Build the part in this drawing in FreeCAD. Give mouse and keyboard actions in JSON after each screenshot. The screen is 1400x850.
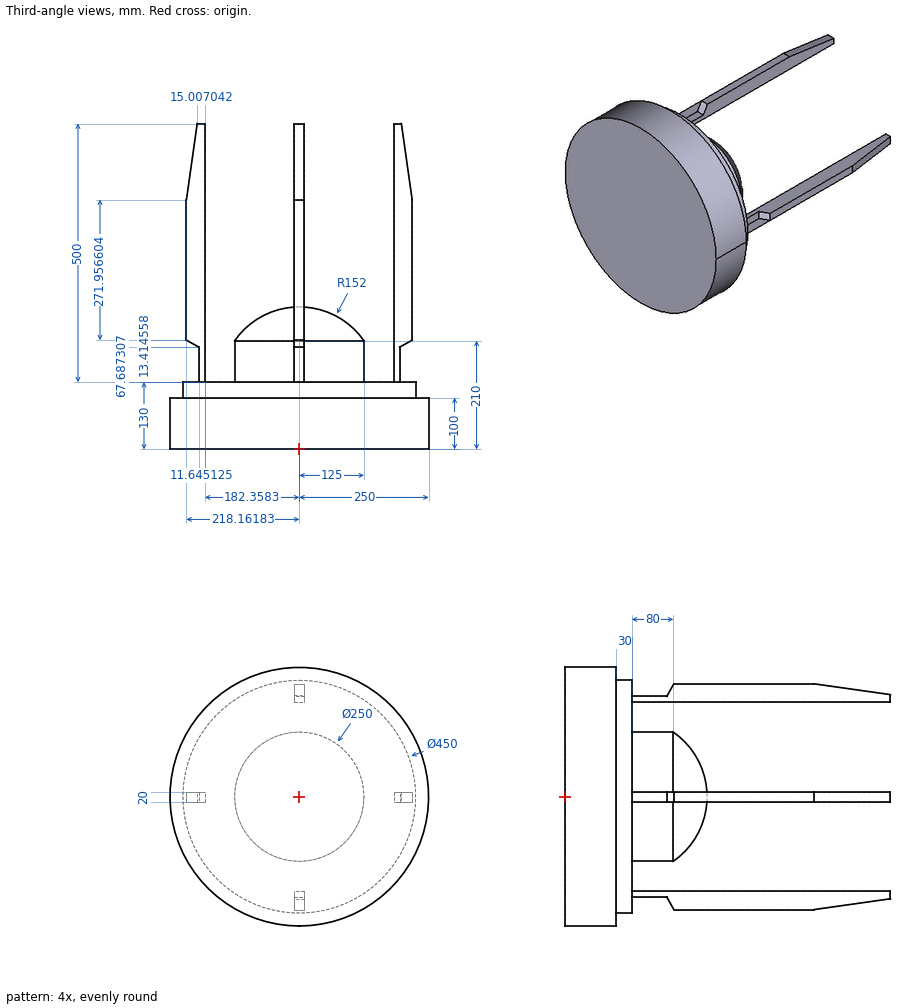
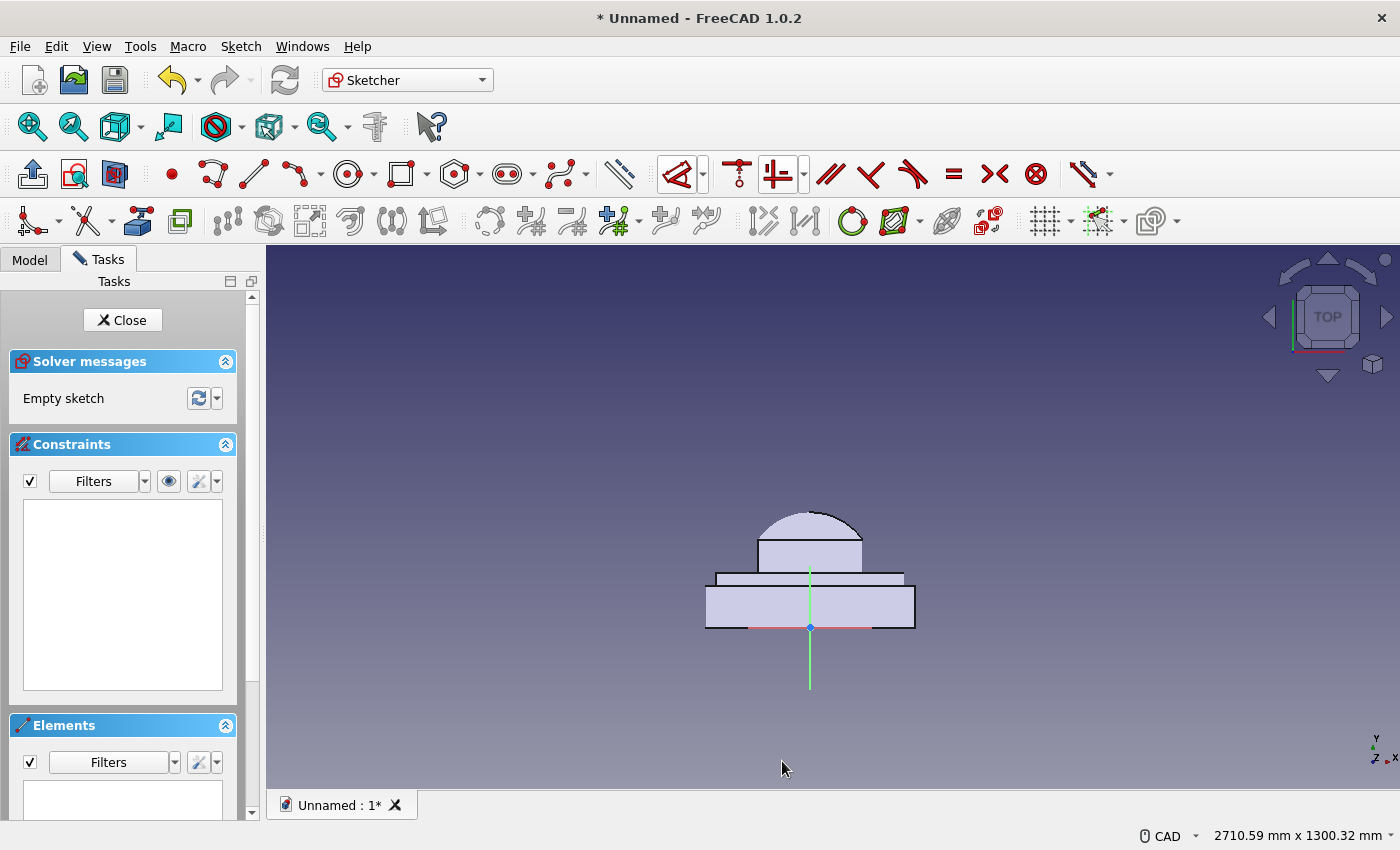
{"action": "left_click", "coordinate": [213, 174]}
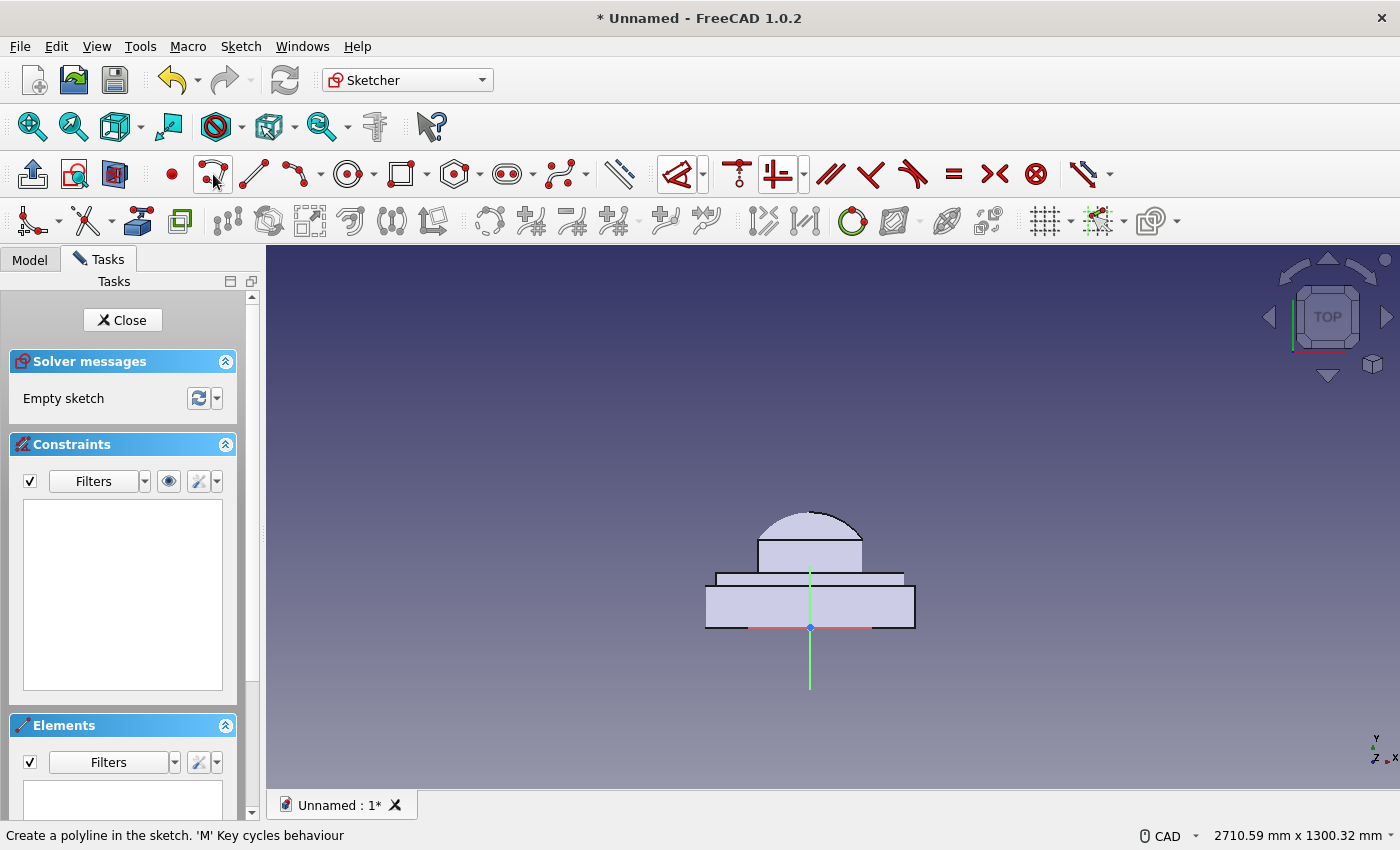
{"action": "left_click", "coordinate": [734, 573]}
{"action": "left_click", "coordinate": [734, 364]}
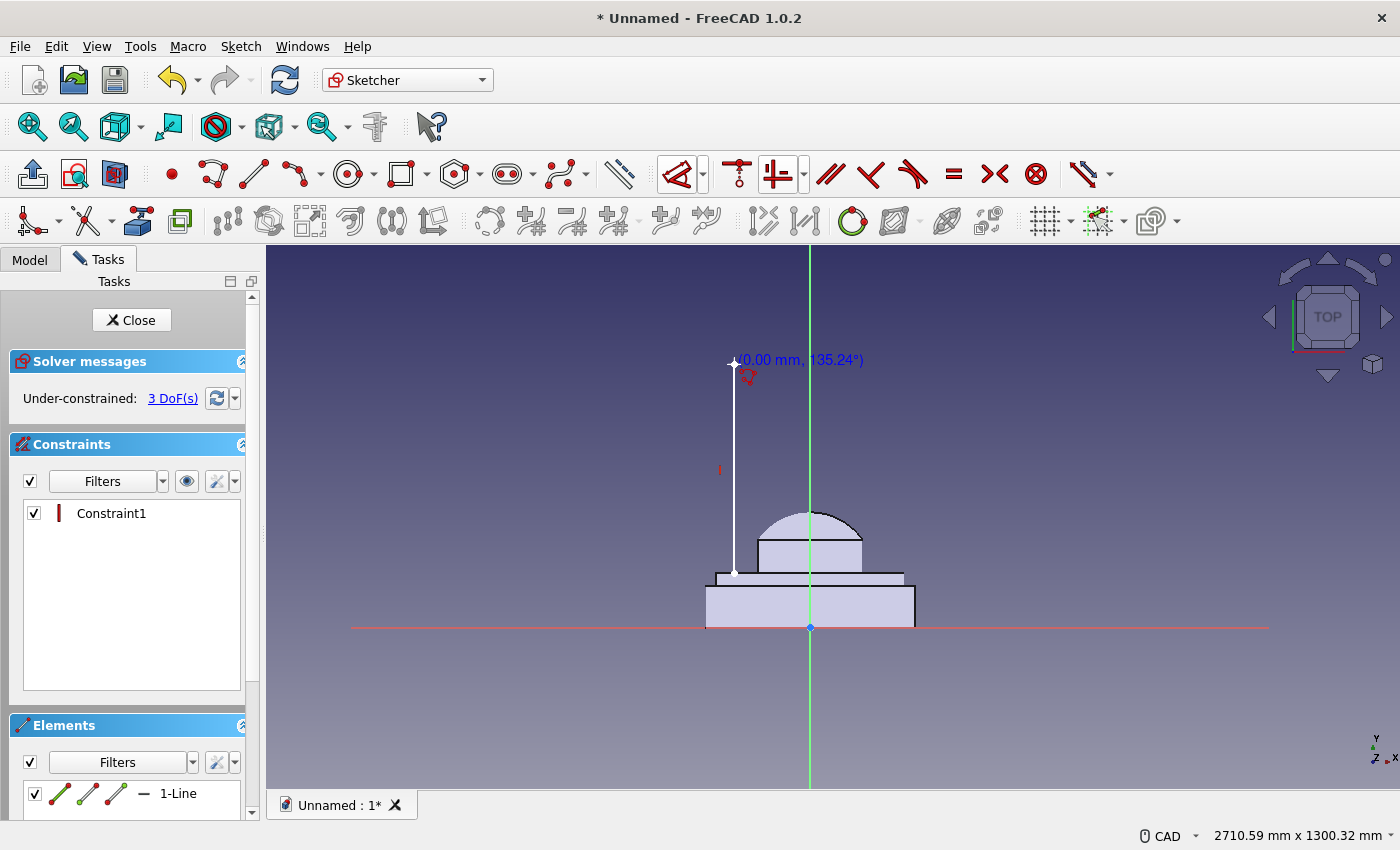
{"action": "scroll", "coordinate": [728, 364], "scroll_direction": "up", "scroll_amount": 5}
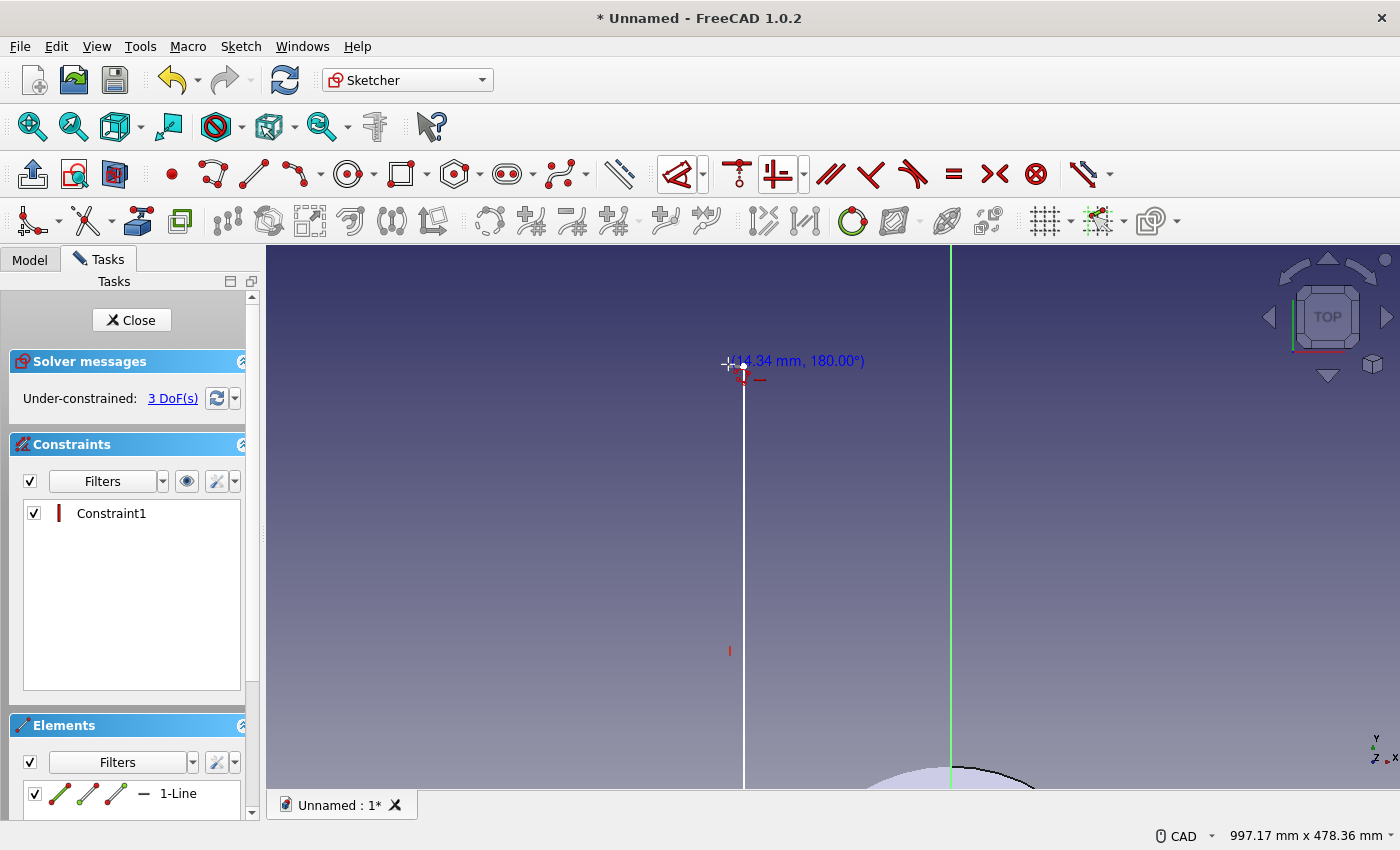
{"action": "left_click", "coordinate": [726, 364]}
{"action": "left_click", "coordinate": [703, 531]}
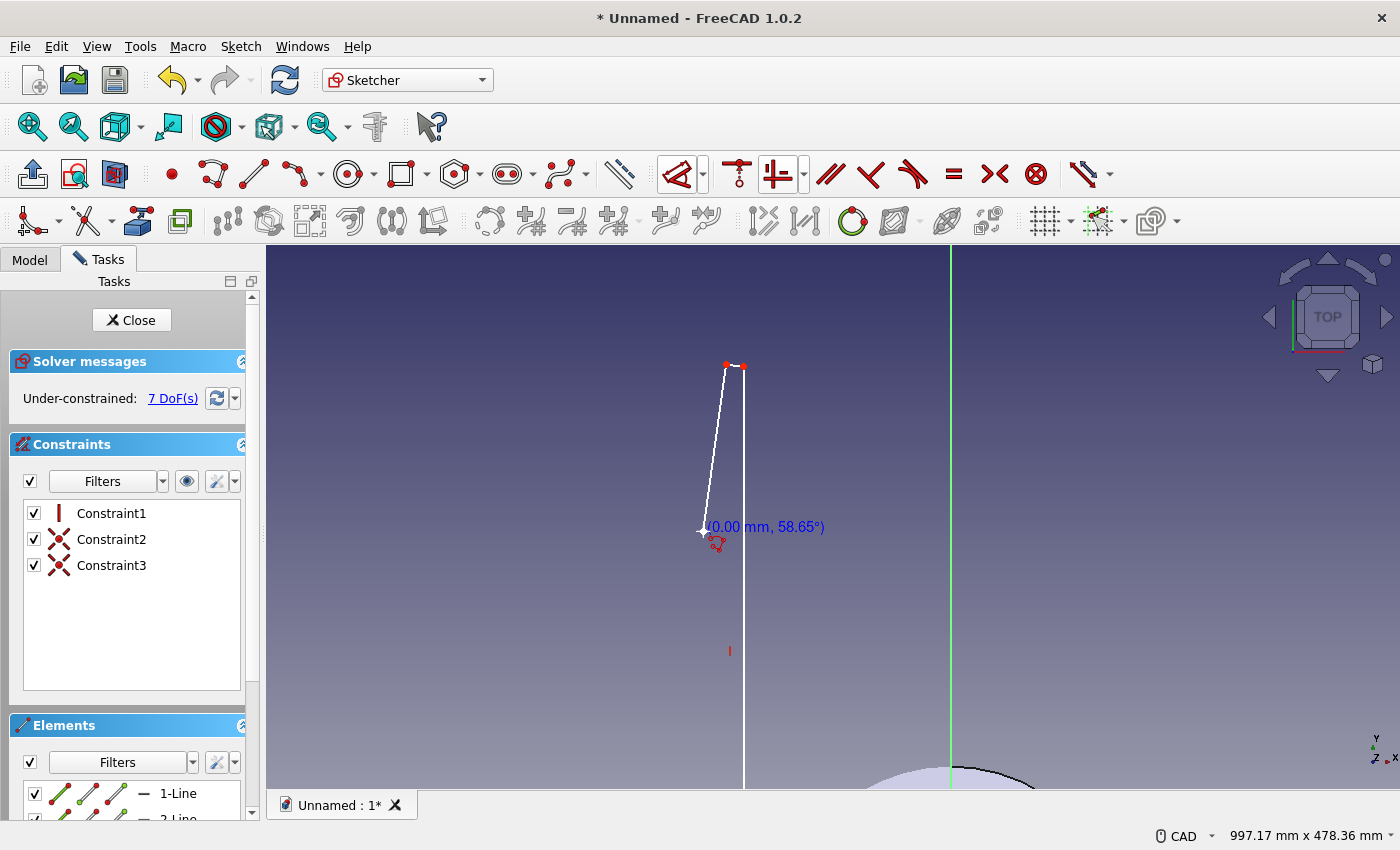
{"action": "scroll", "coordinate": [714, 350], "scroll_direction": "down", "scroll_amount": 4}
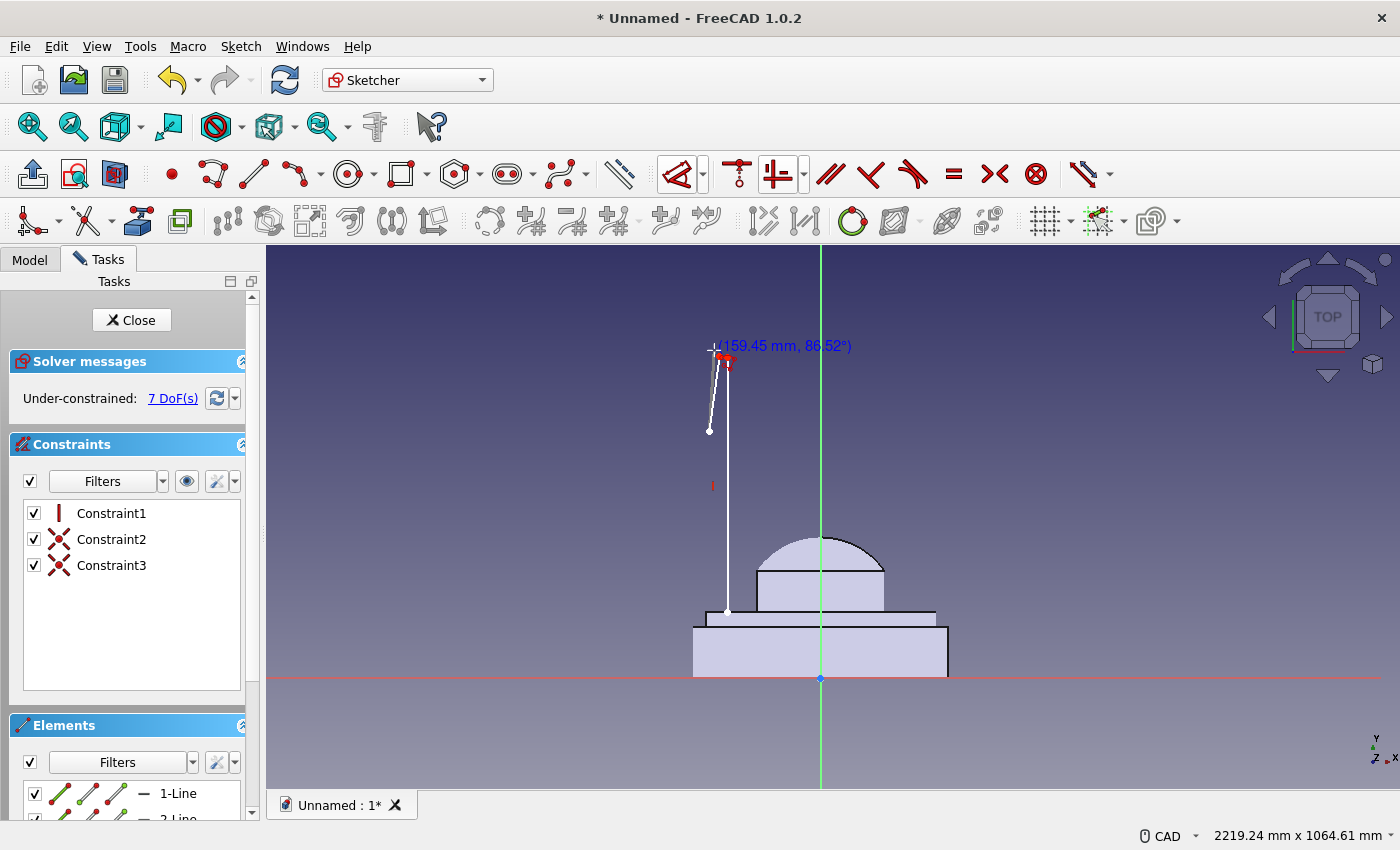
{"action": "left_click", "coordinate": [709, 570]}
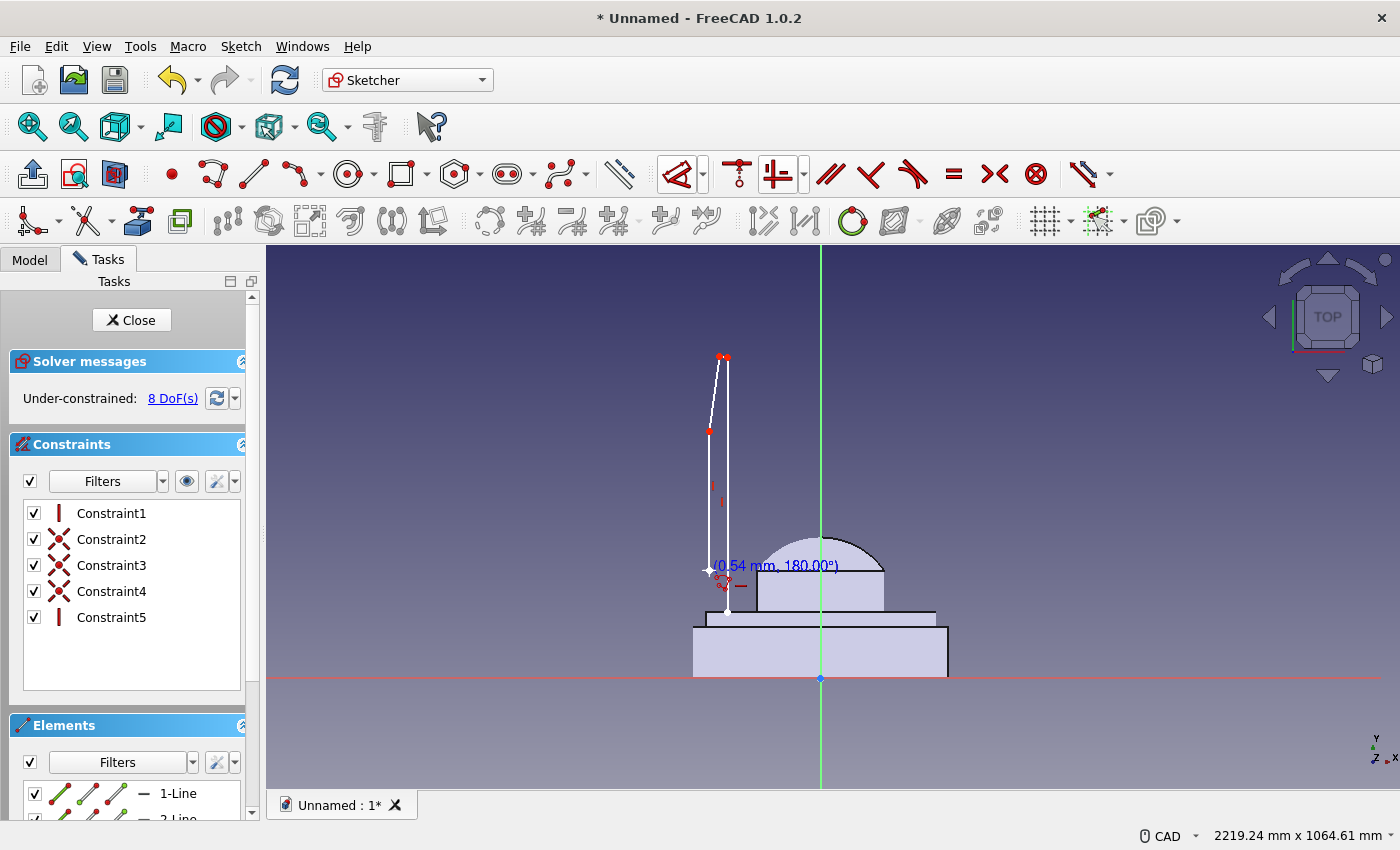
{"action": "scroll", "coordinate": [721, 577], "scroll_direction": "up", "scroll_amount": 5}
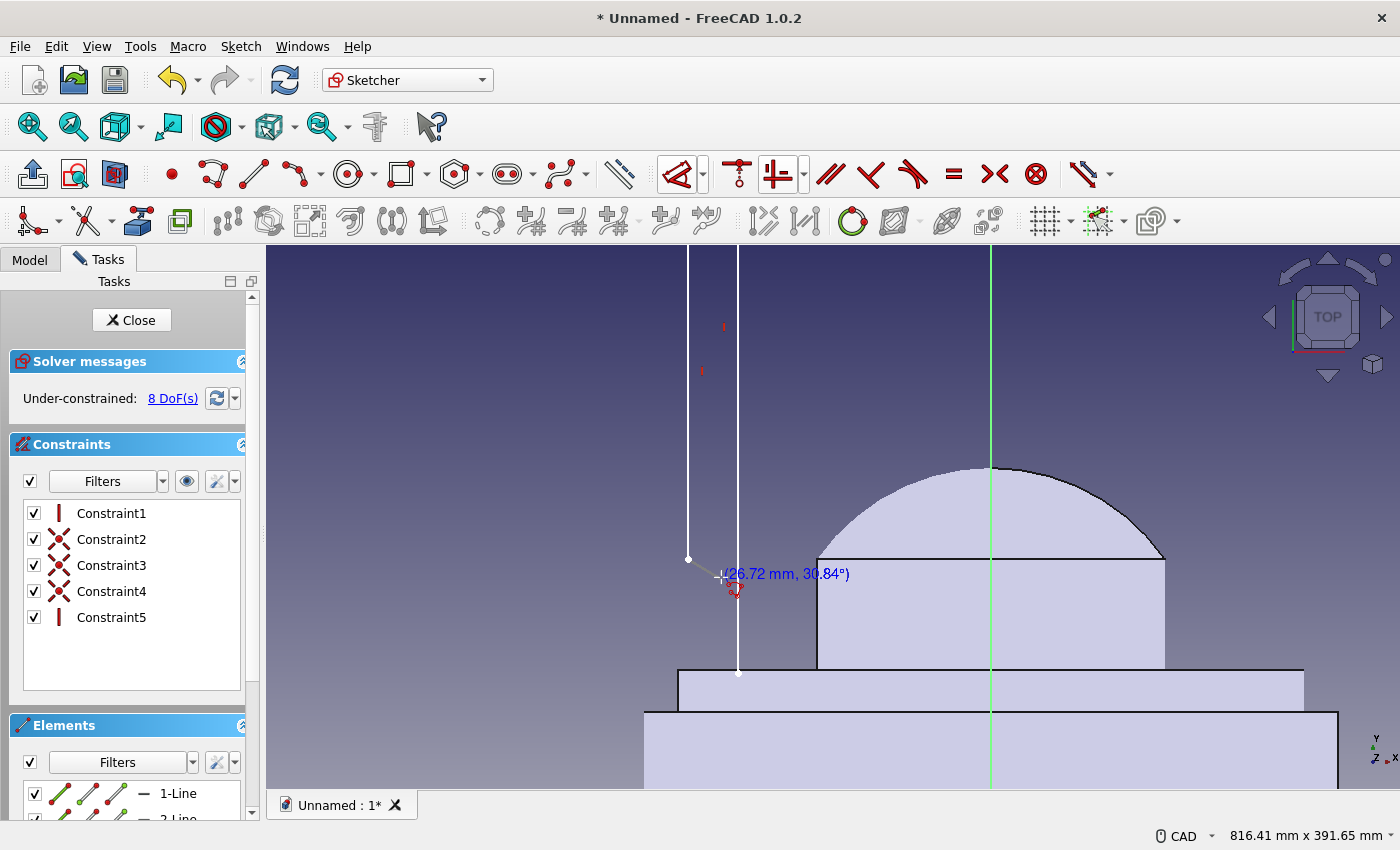
{"action": "left_click", "coordinate": [722, 576]}
{"action": "left_click", "coordinate": [722, 670]}
{"action": "left_click", "coordinate": [738, 673]}
{"action": "key", "text": "Escape"}
{"action": "key", "text": "Escape"}